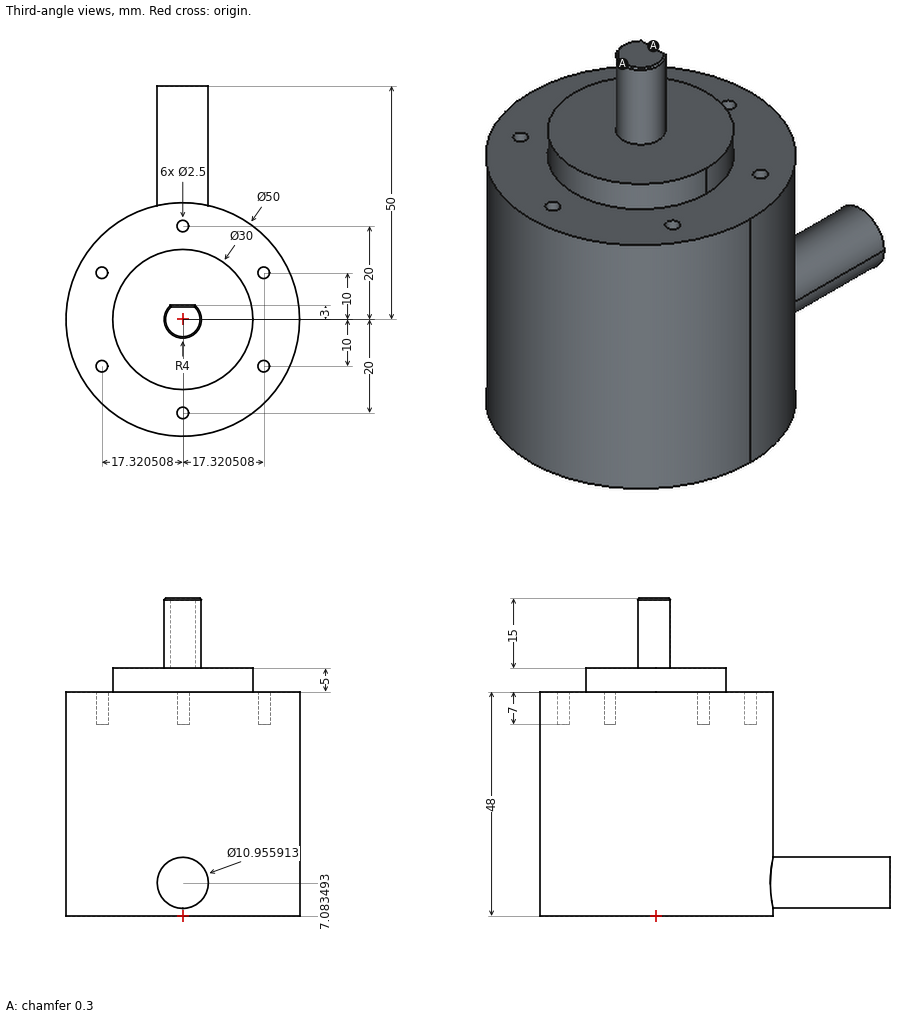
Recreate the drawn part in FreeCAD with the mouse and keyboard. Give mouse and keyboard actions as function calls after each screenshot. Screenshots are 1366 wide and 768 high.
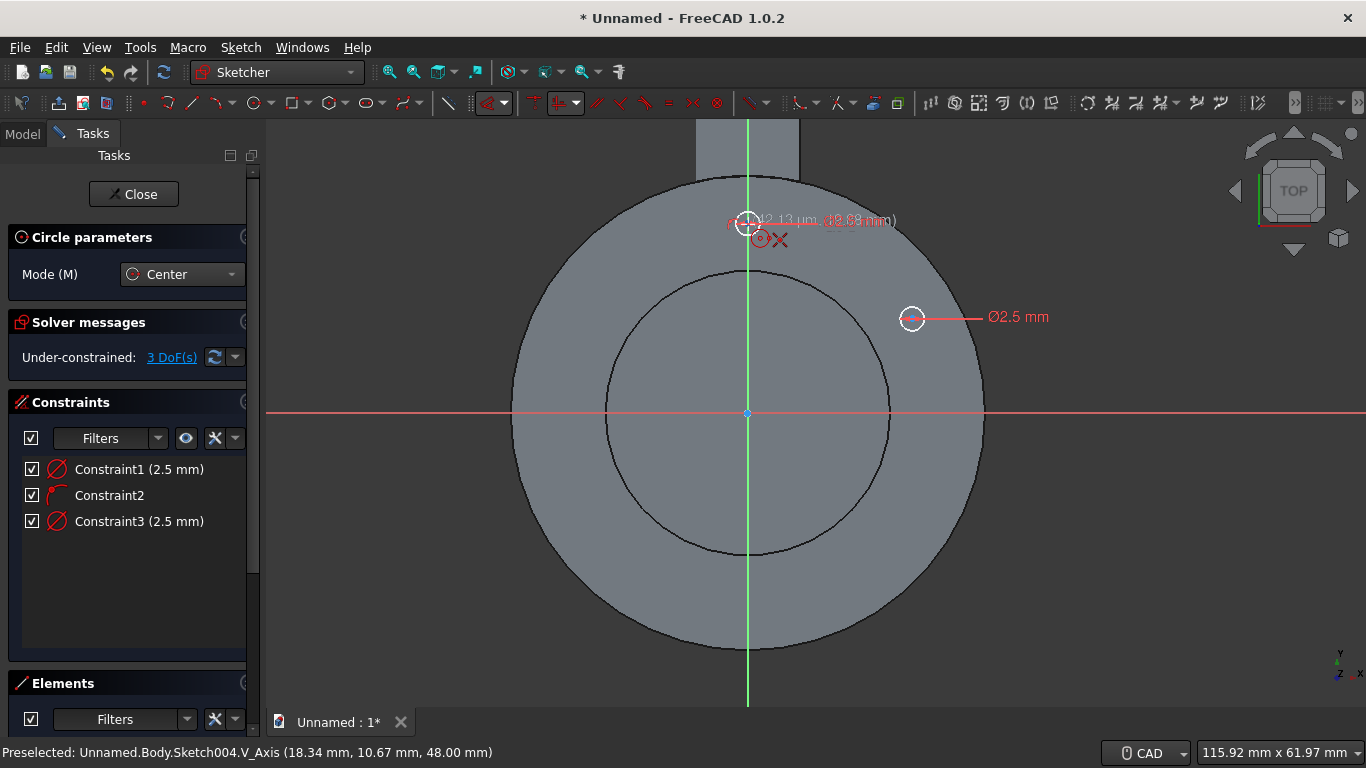
scroll(912, 508, up, 4)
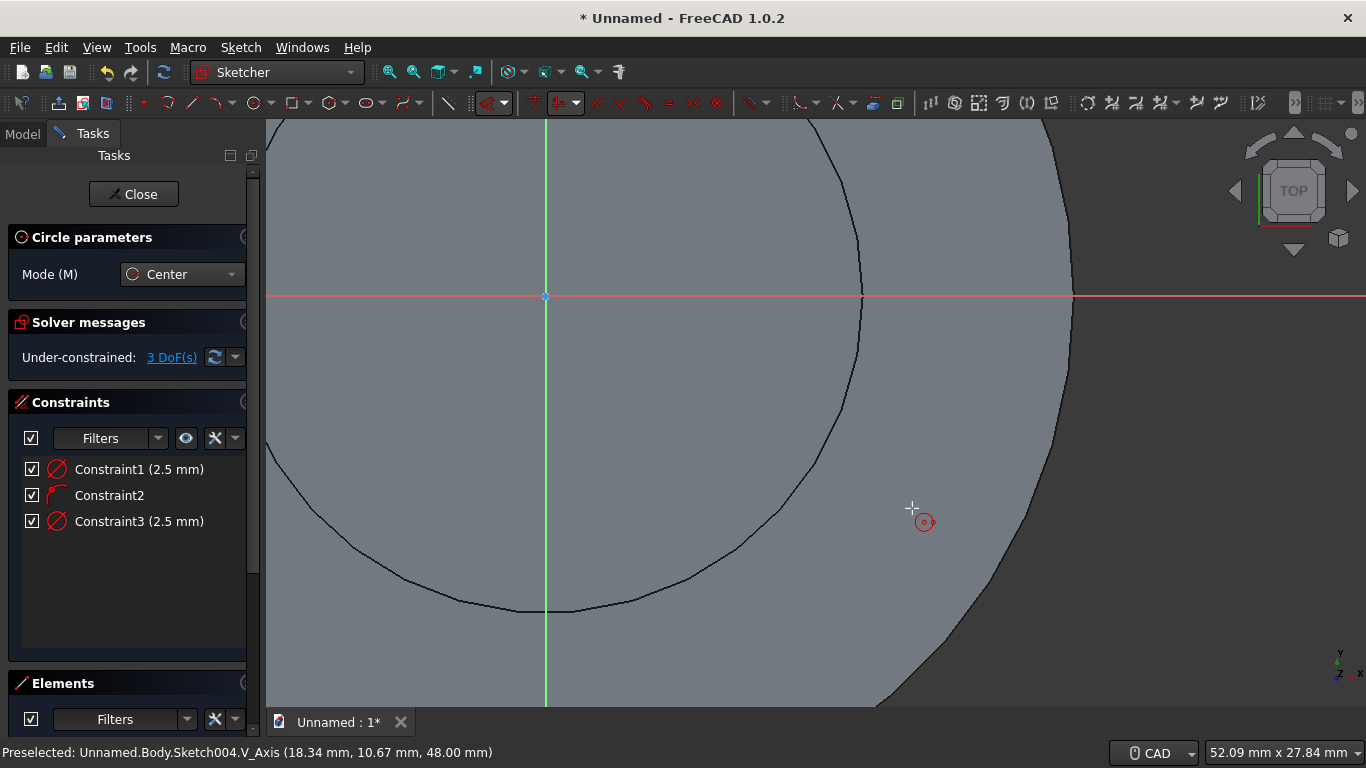
click(912, 507)
move(930, 489)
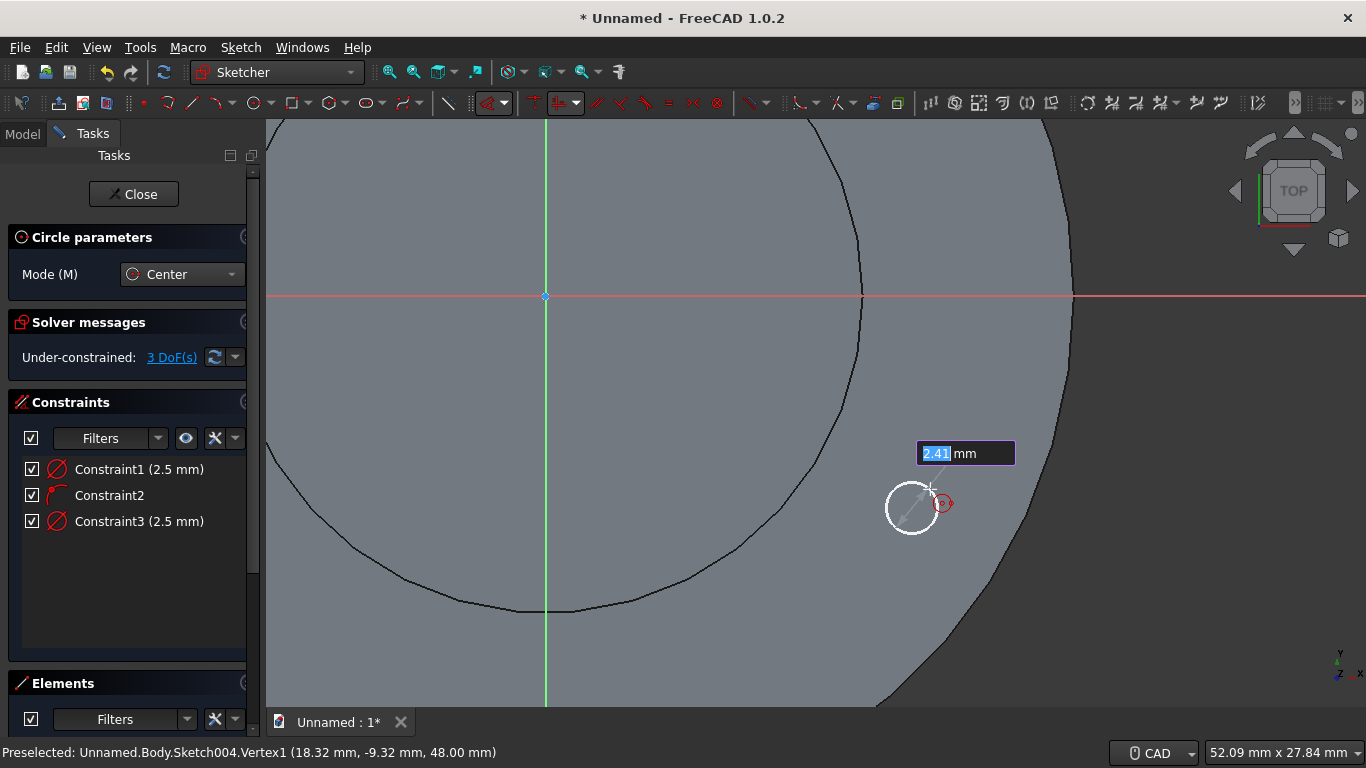
text(2.5)
key(Return)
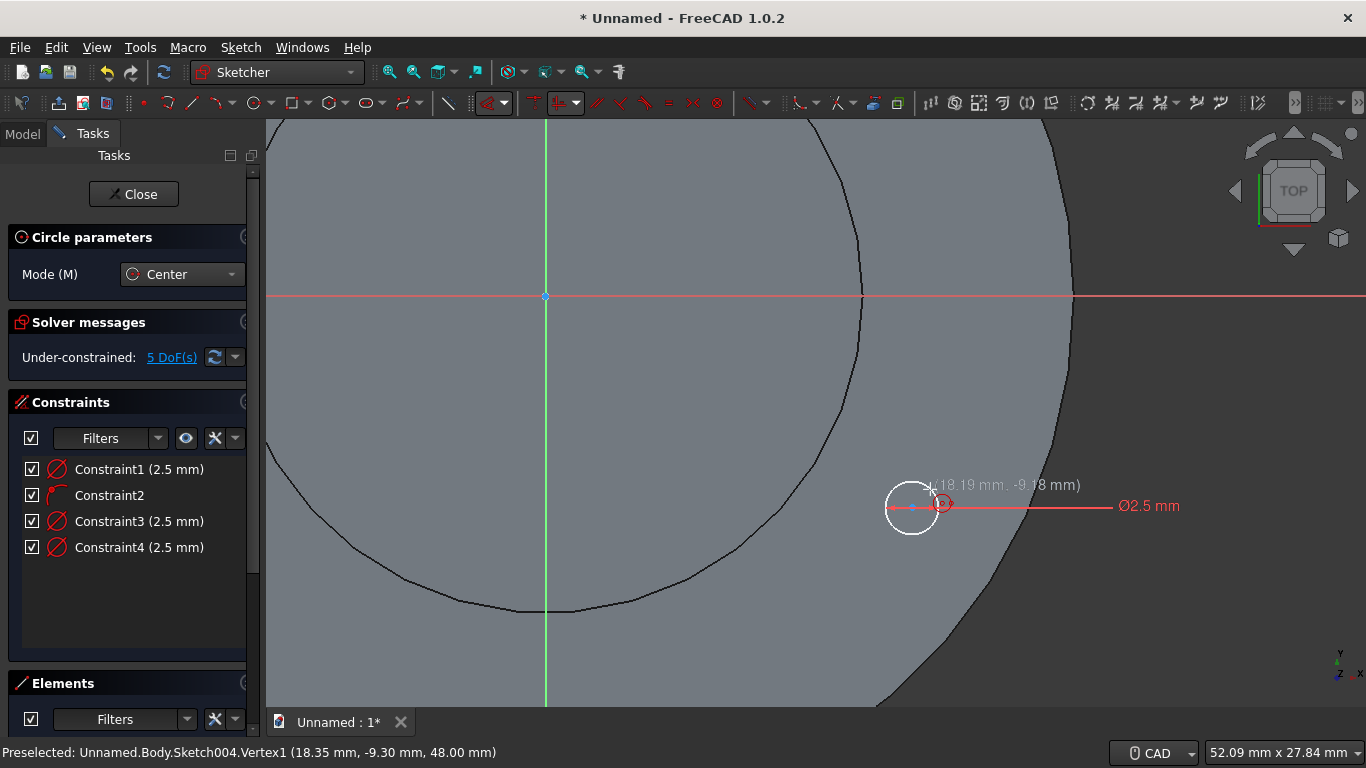
scroll(912, 508, down, 4)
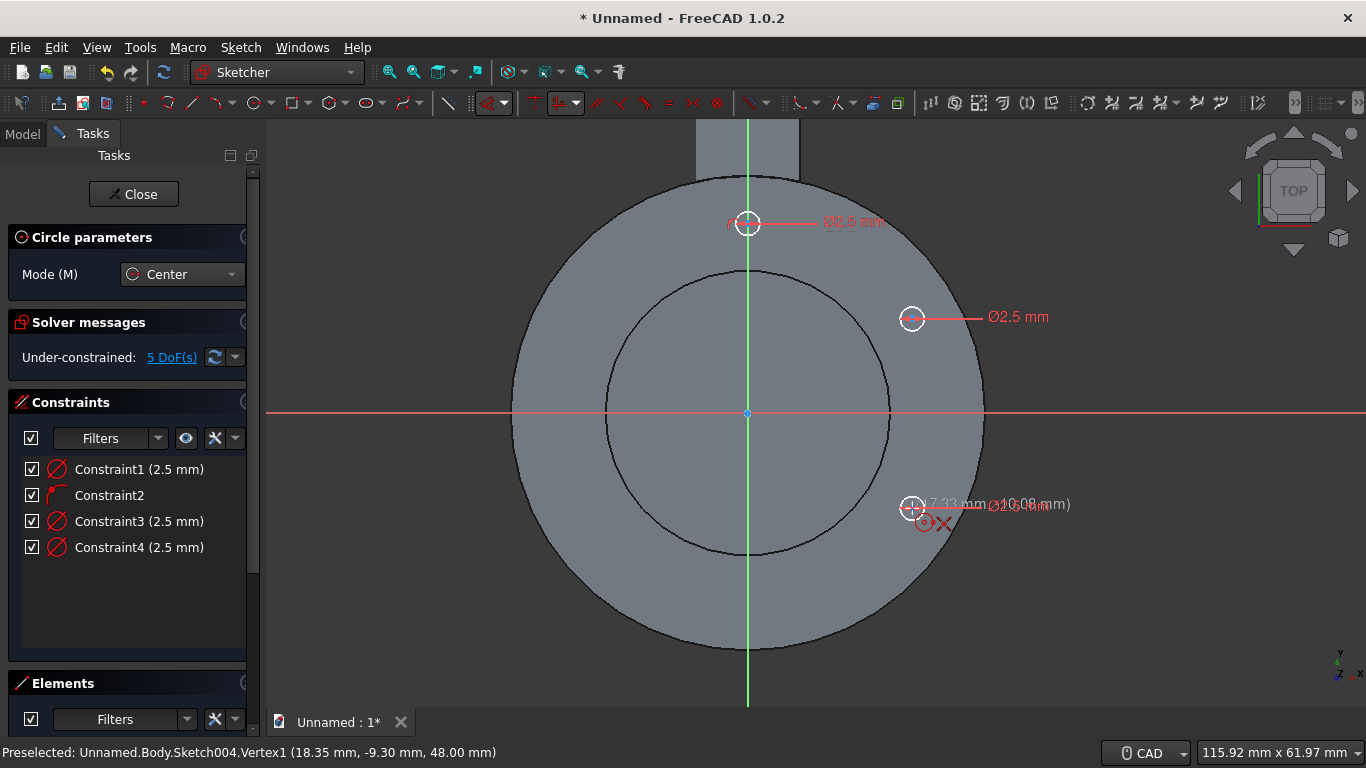
scroll(748, 603, up, 4)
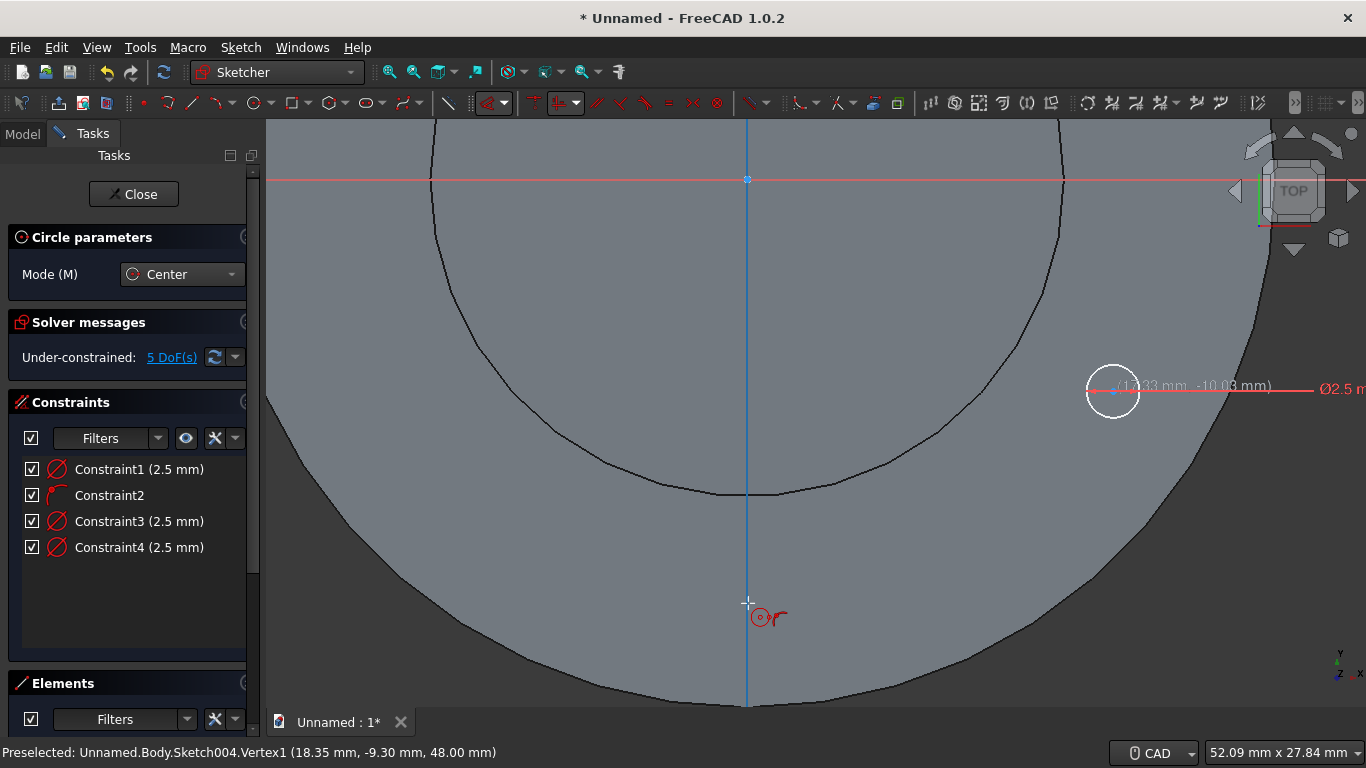
click(747, 602)
move(766, 583)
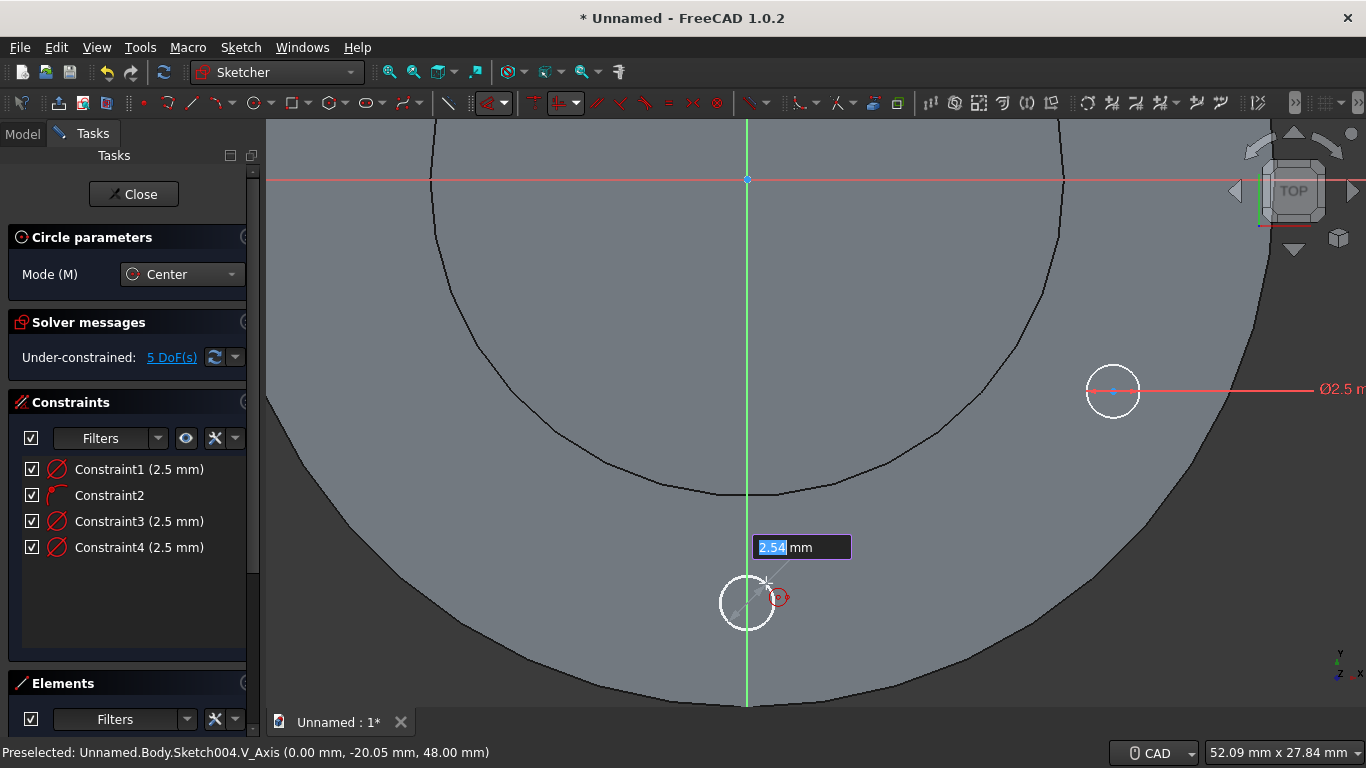
text(2.5)
key(Return)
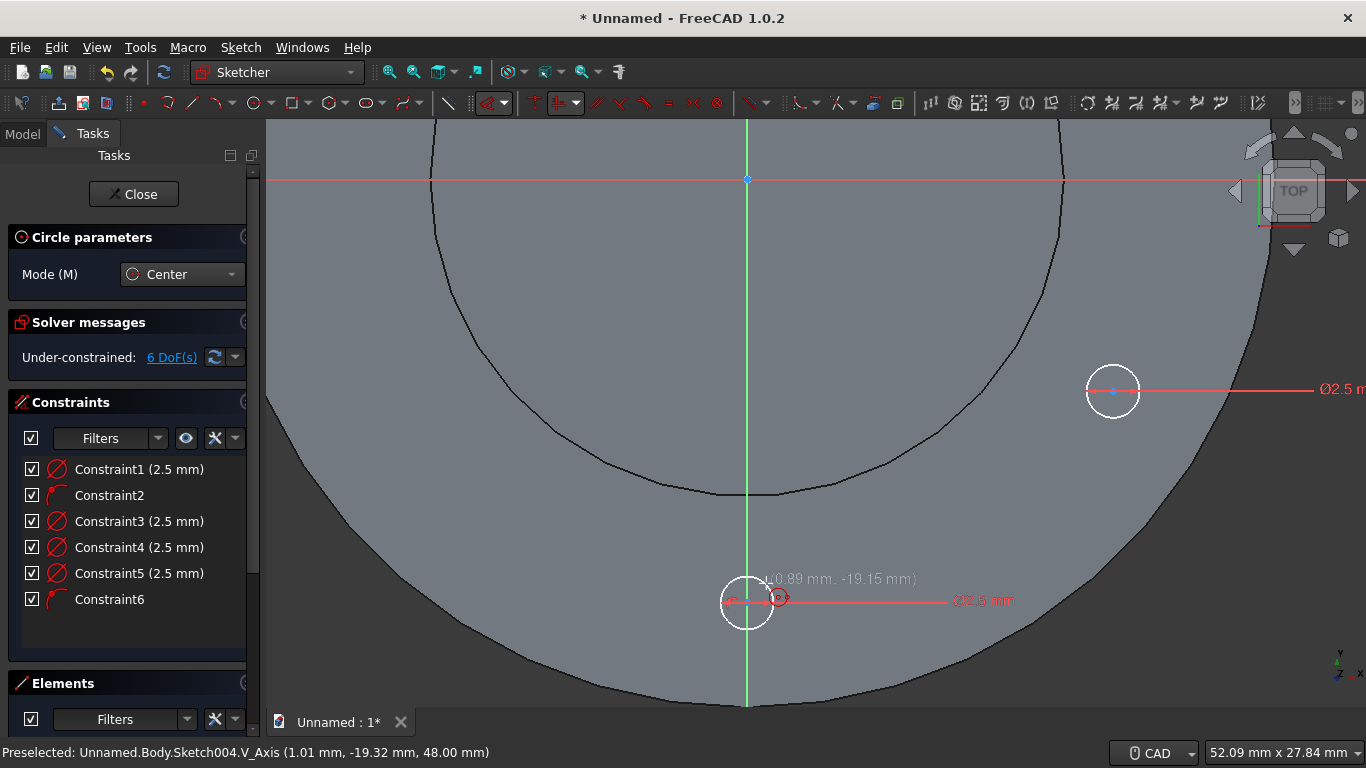
click(381, 391)
move(400, 372)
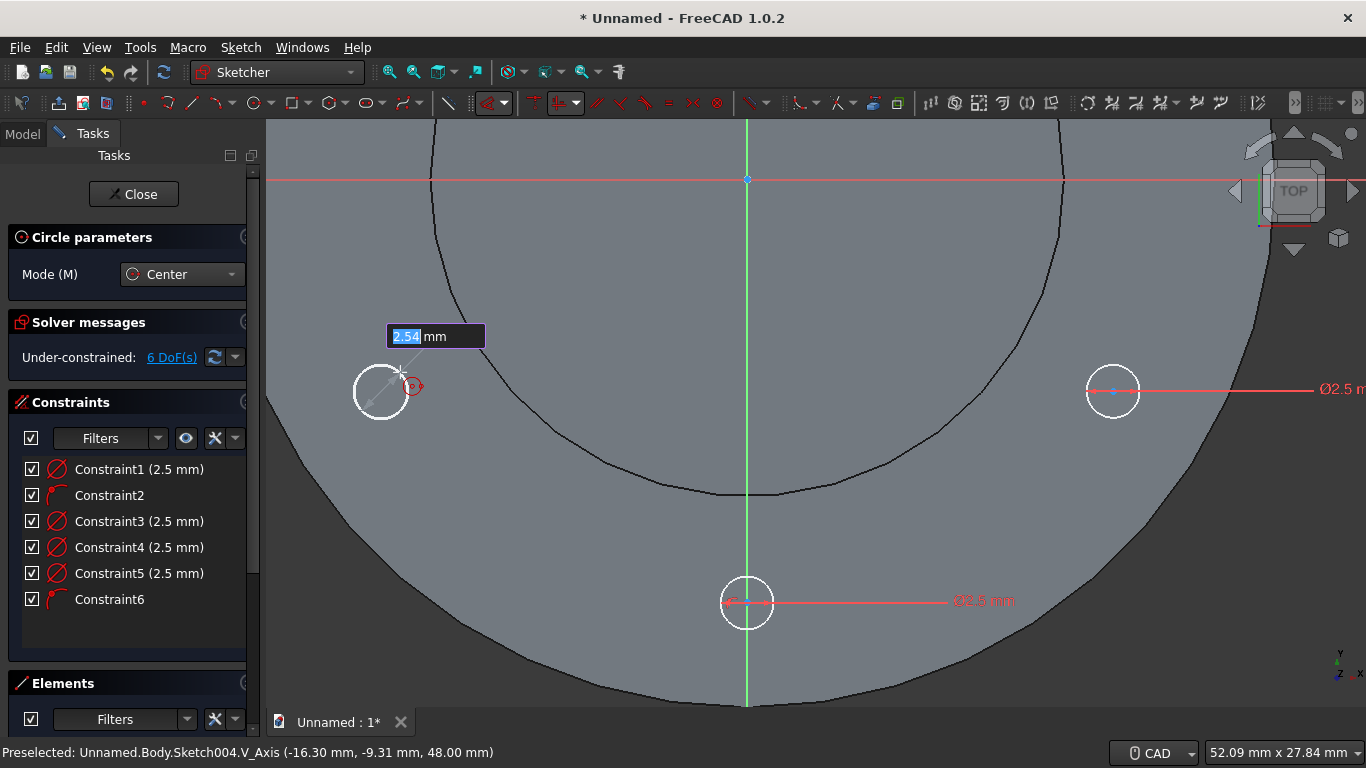
text(2.5)
key(Return)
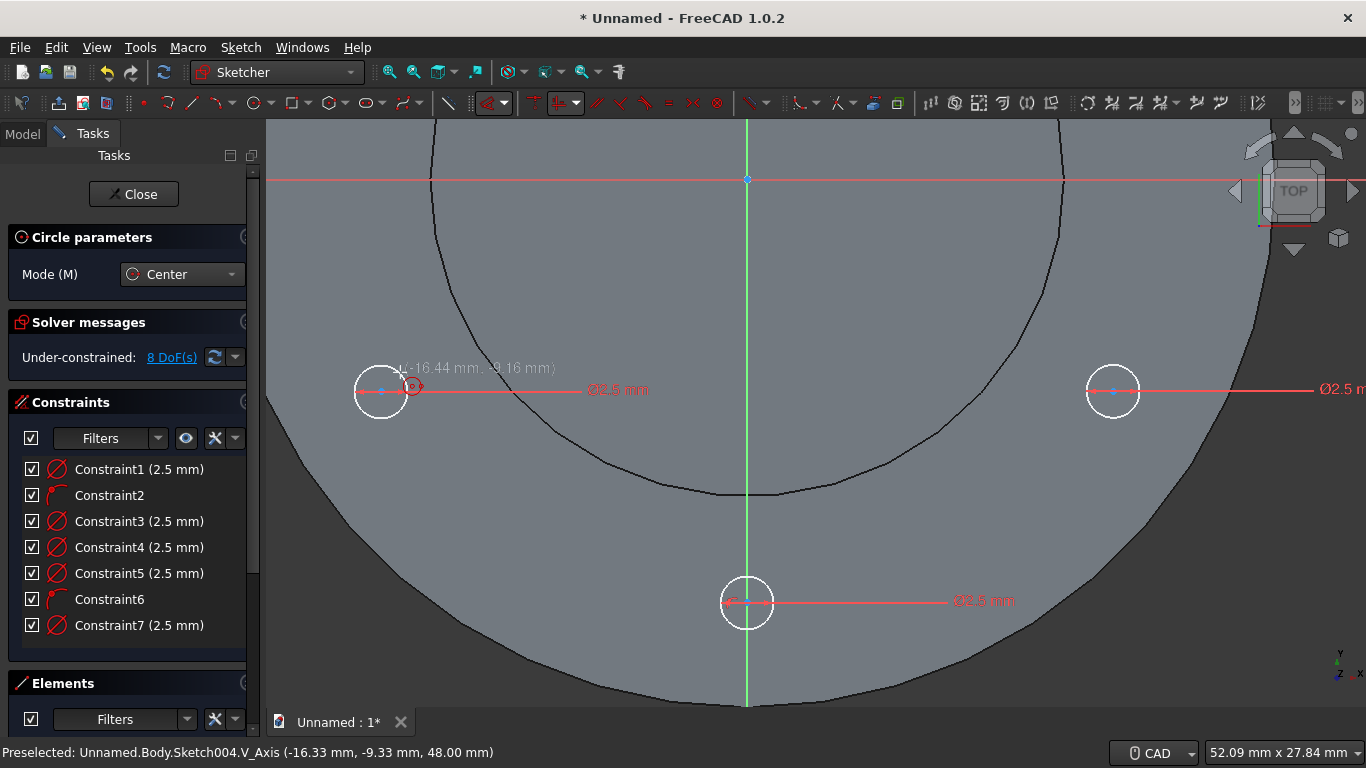
scroll(748, 604, down, 4)